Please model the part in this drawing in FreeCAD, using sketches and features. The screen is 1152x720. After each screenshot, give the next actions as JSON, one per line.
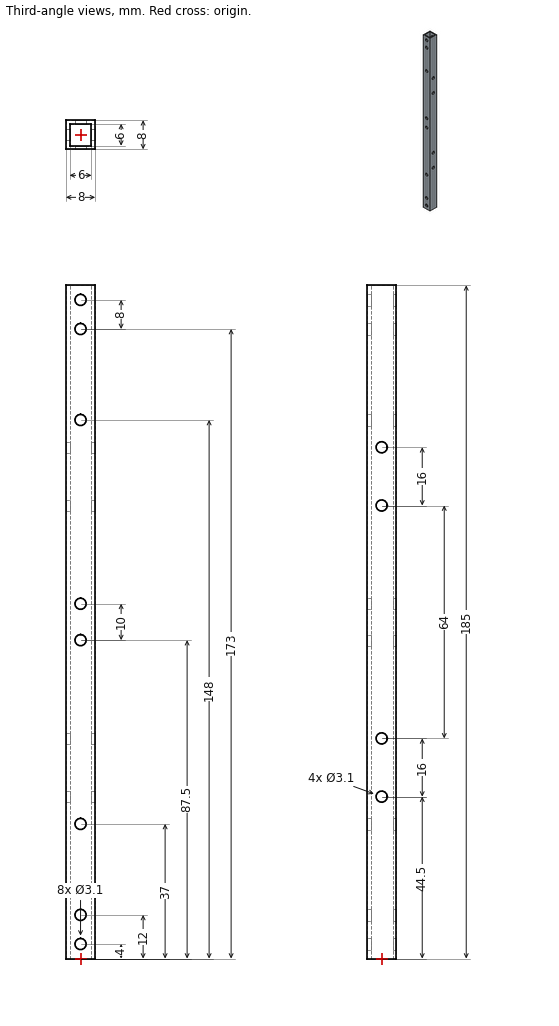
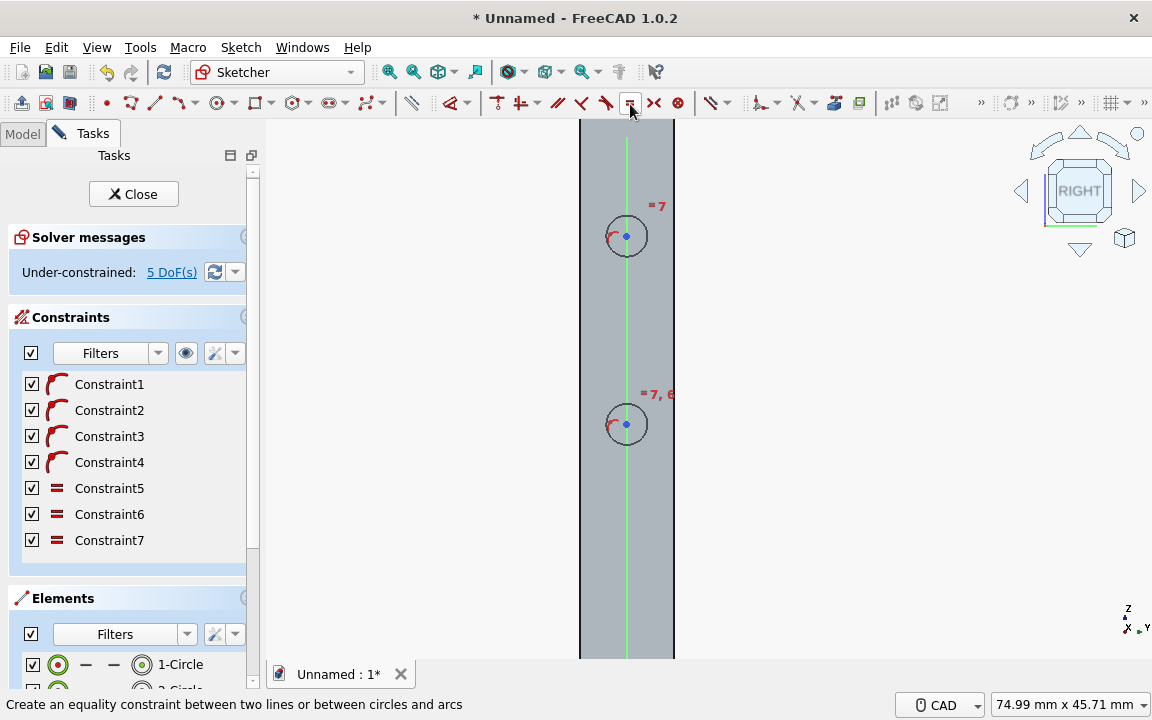
{"action": "left_click", "coordinate": [450, 104]}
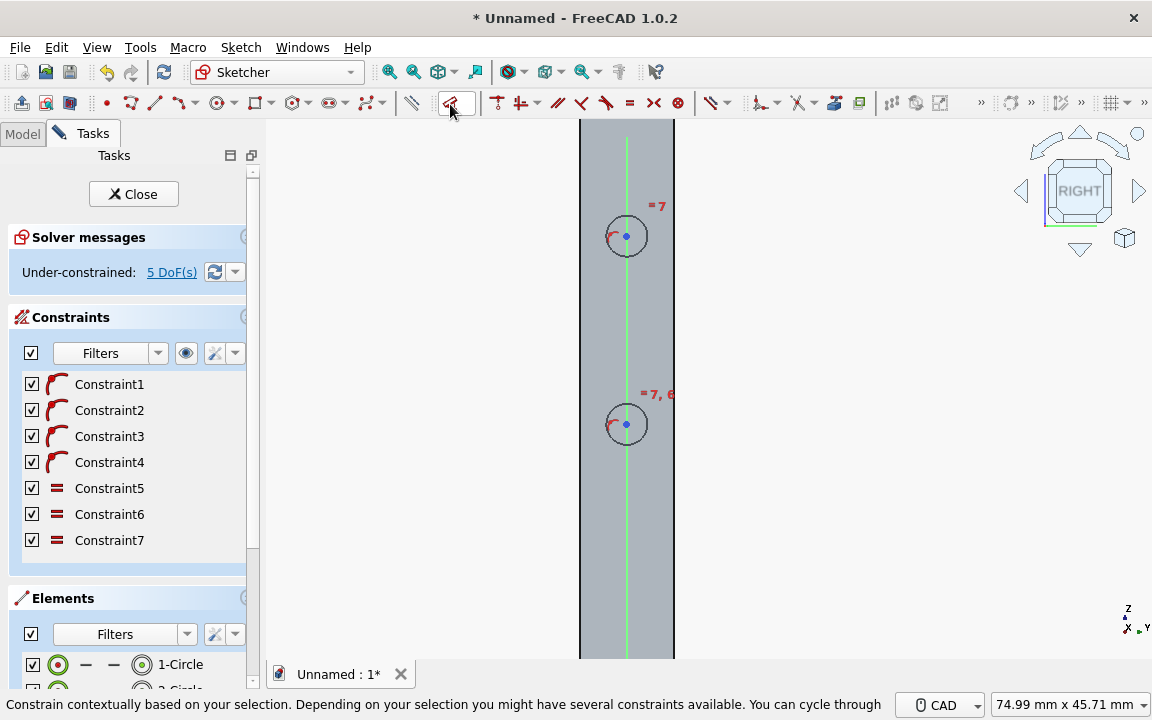
{"action": "scroll", "coordinate": [644, 222], "scroll_direction": "down", "scroll_amount": 8}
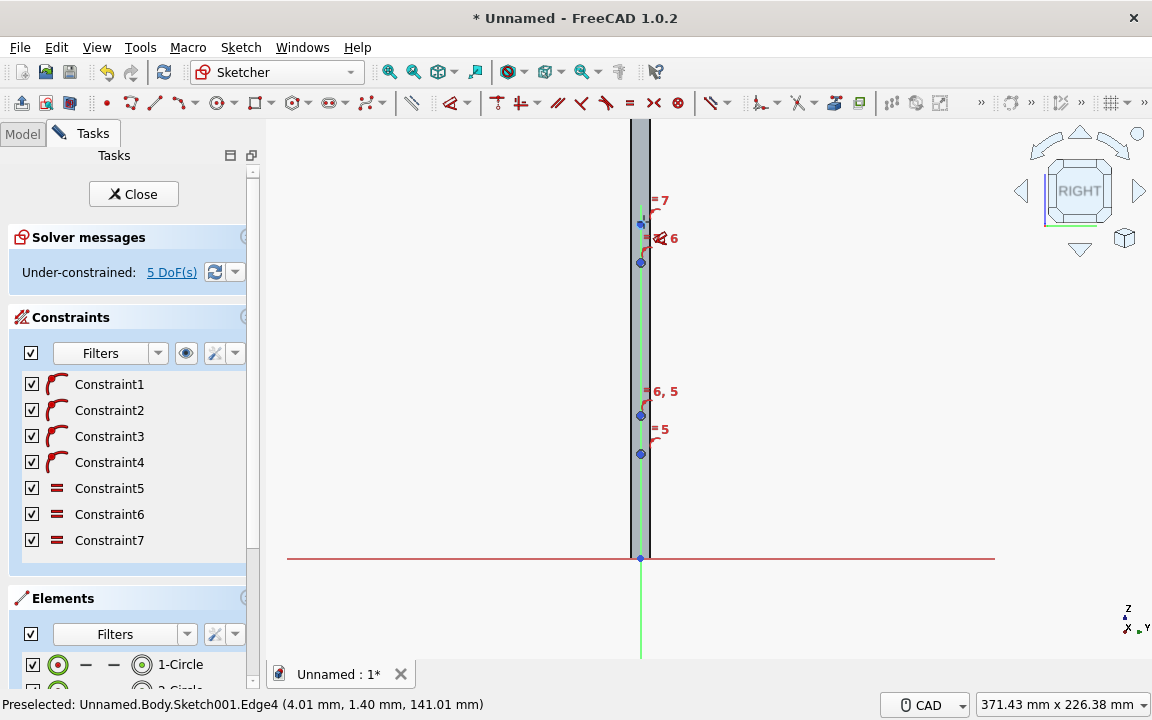
{"action": "scroll", "coordinate": [644, 451], "scroll_direction": "up", "scroll_amount": 9}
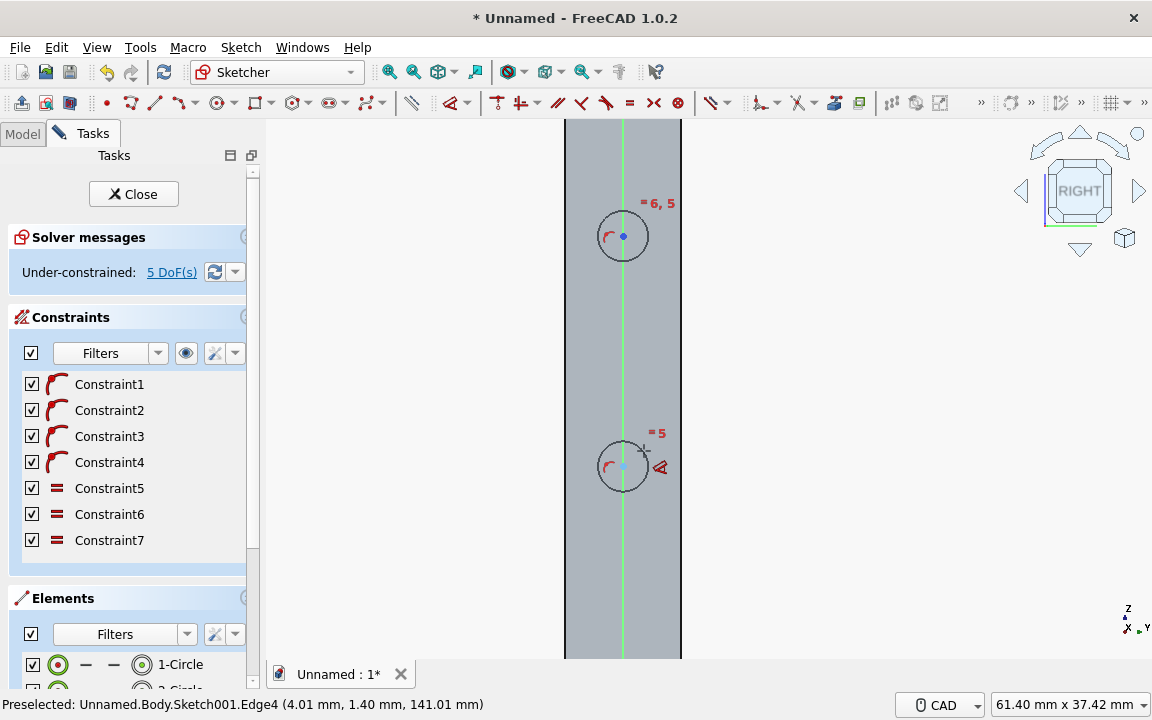
{"action": "left_click", "coordinate": [641, 449]}
{"action": "left_click", "coordinate": [664, 427]}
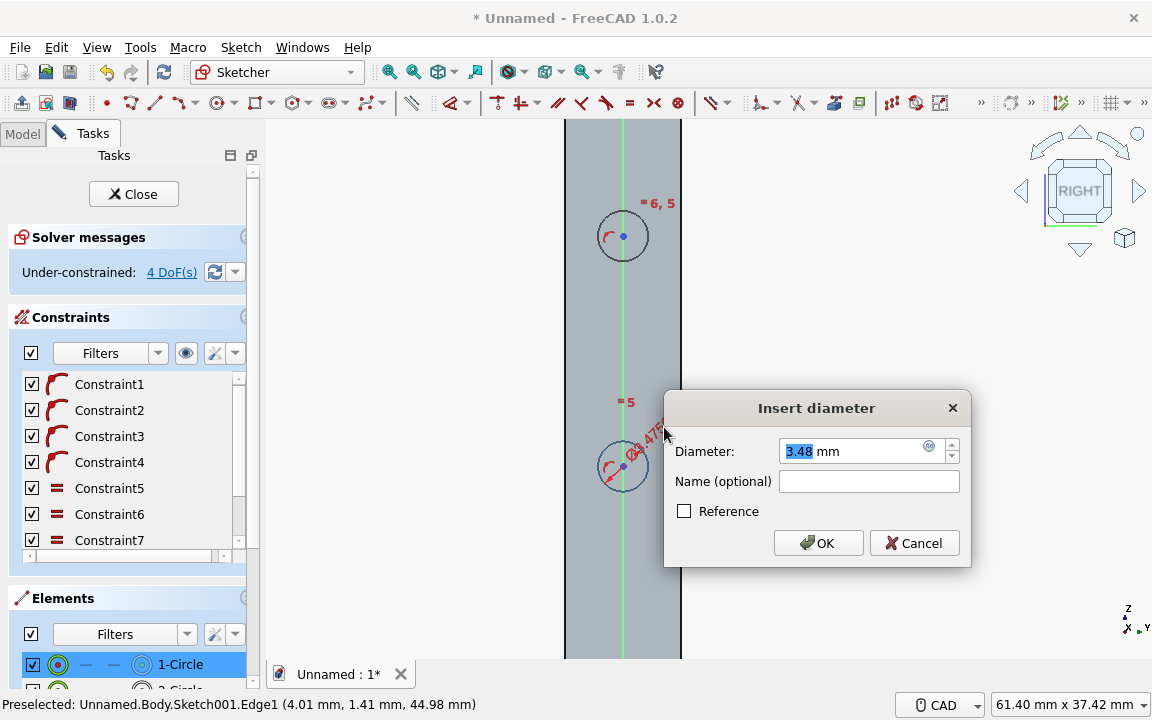
{"action": "type", "text": "3.1"}
{"action": "key", "text": "Return"}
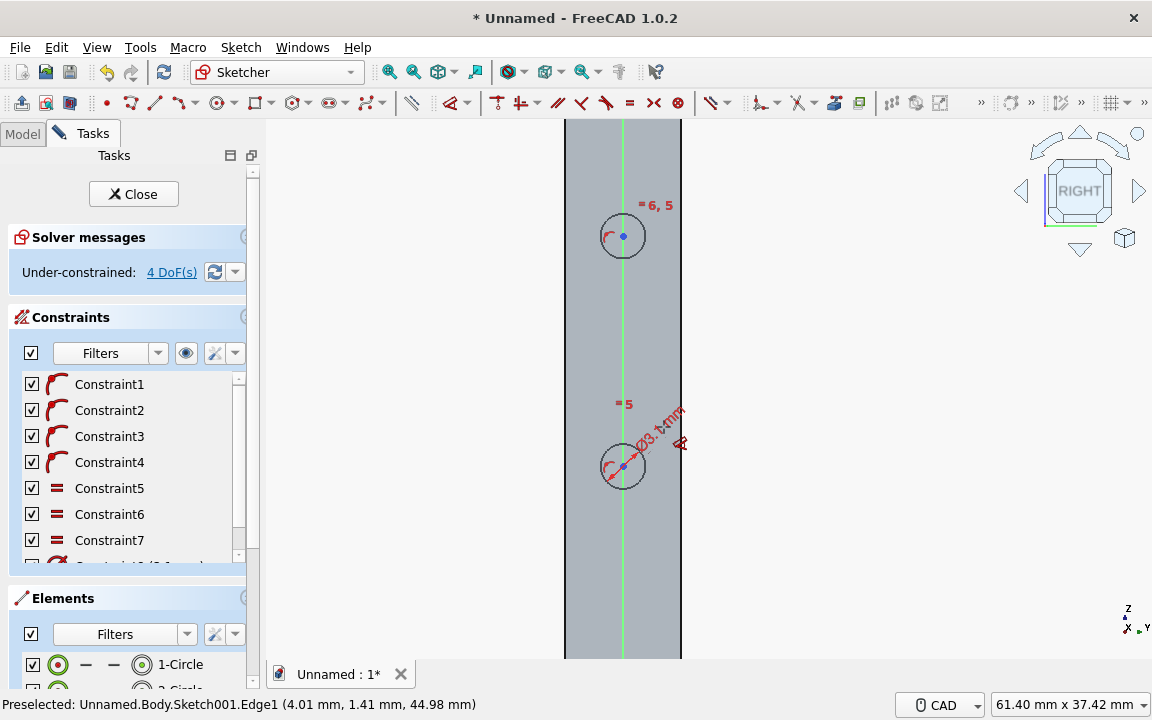
{"action": "scroll", "coordinate": [644, 451], "scroll_direction": "down", "scroll_amount": 9}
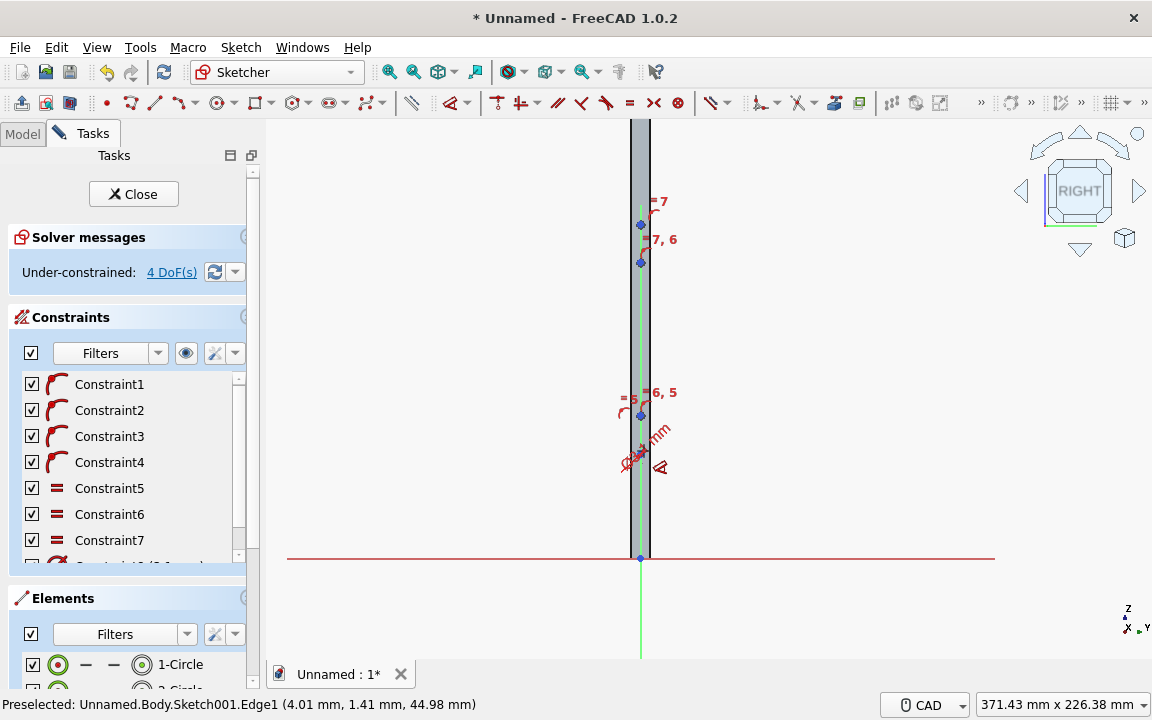
{"action": "left_click", "coordinate": [641, 454]}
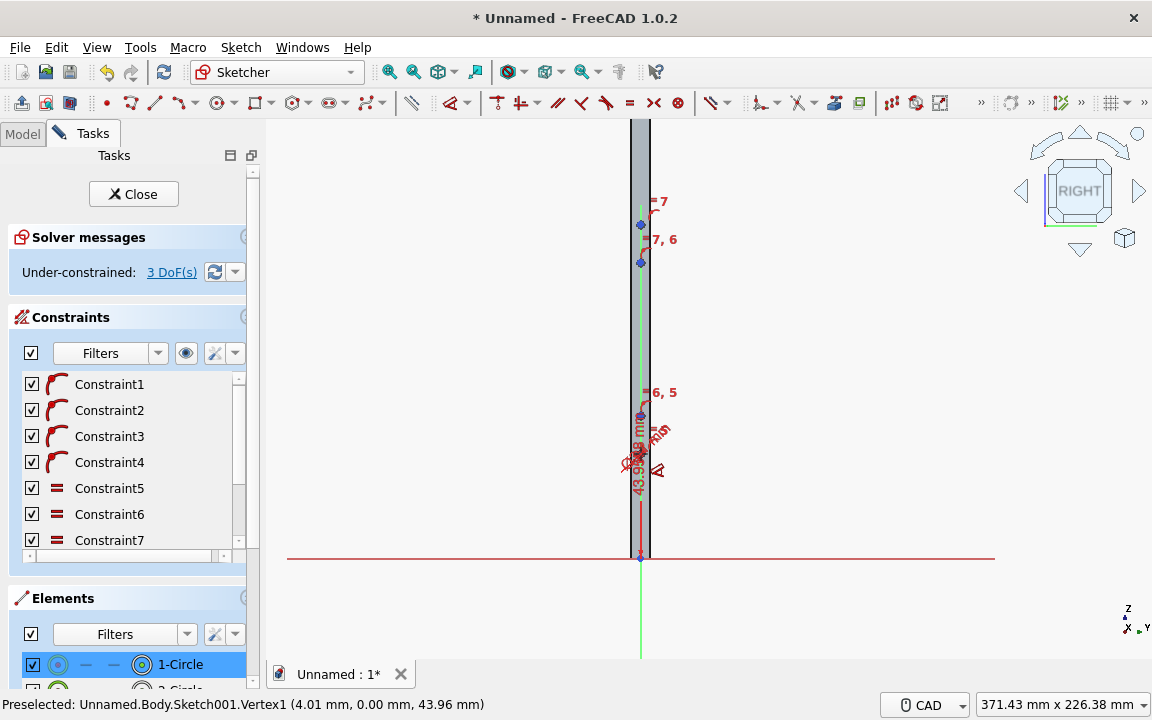
{"action": "left_click", "coordinate": [641, 416]}
{"action": "left_click", "coordinate": [675, 426]}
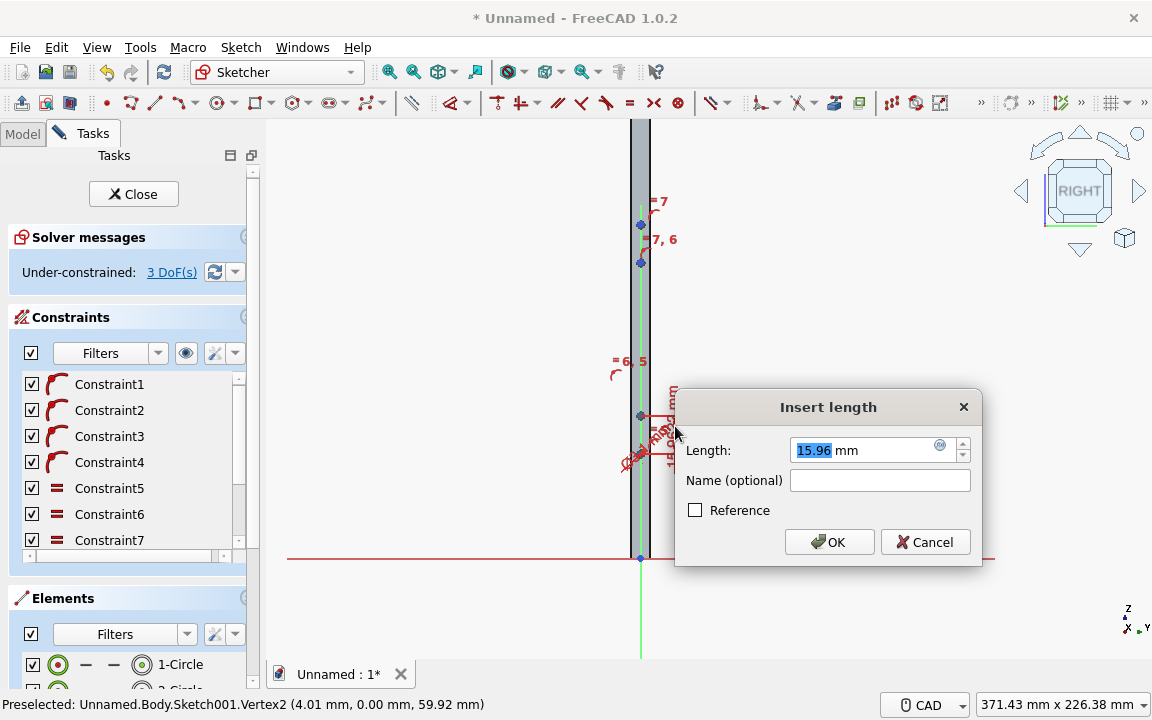
{"action": "type", "text": "16"}
{"action": "key", "text": "Return"}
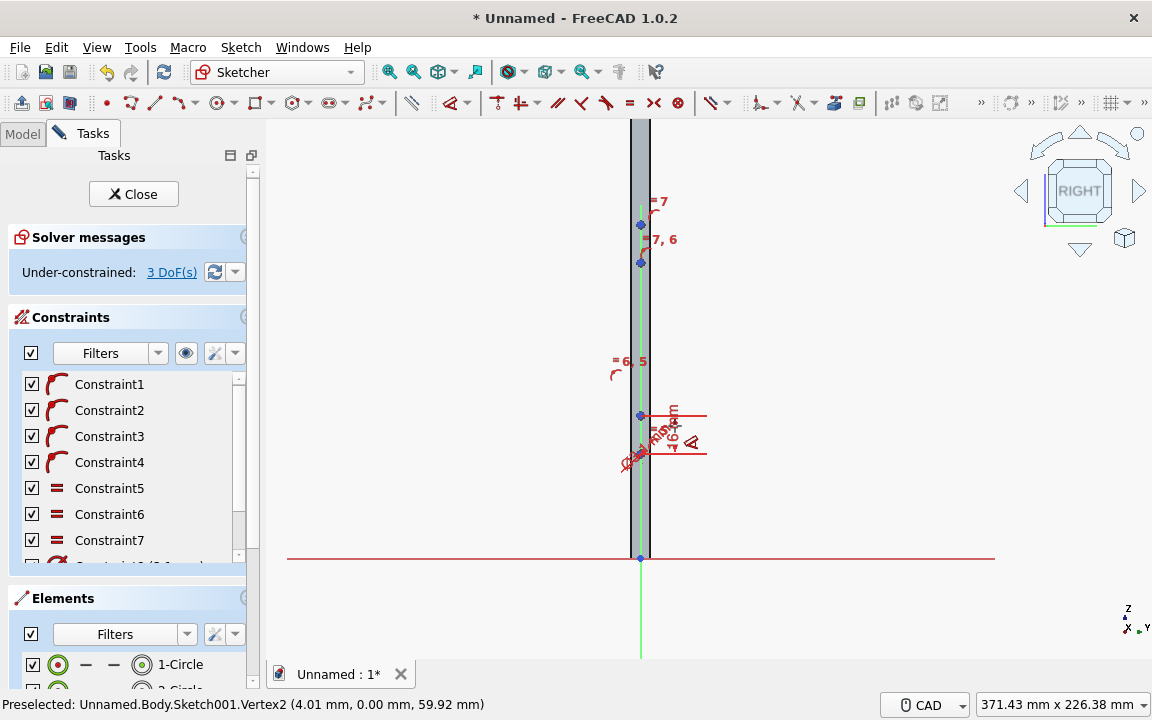
{"action": "left_click", "coordinate": [641, 416]}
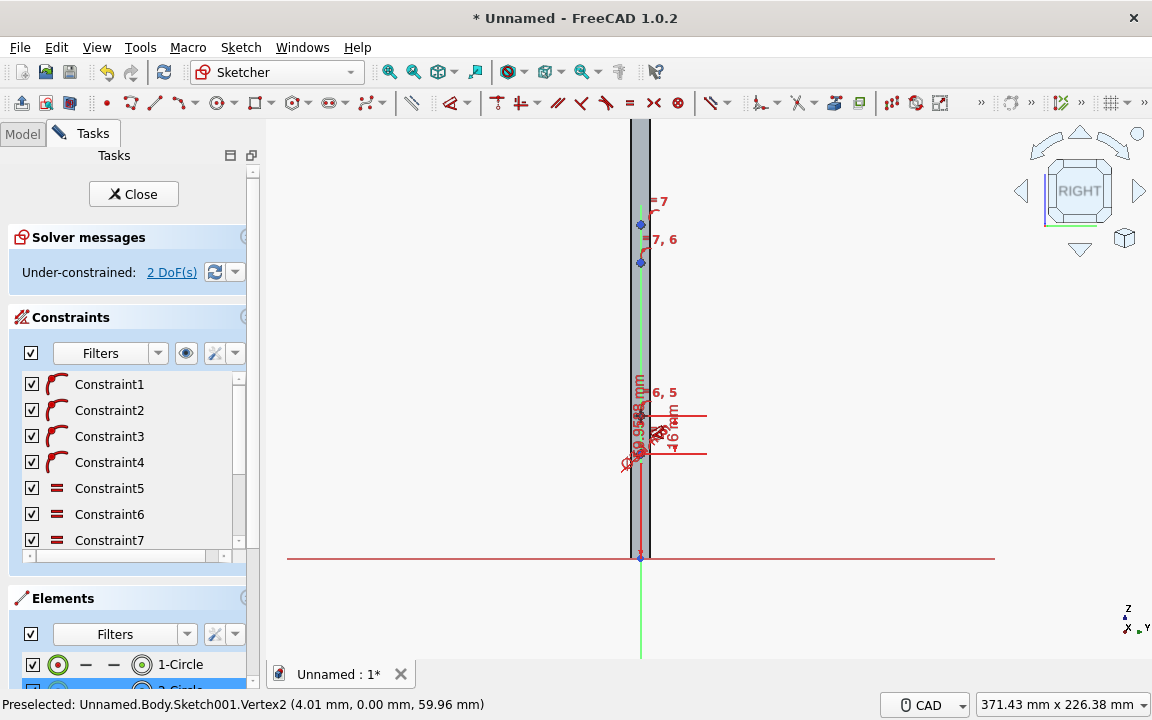
{"action": "left_click", "coordinate": [641, 263]}
{"action": "left_click", "coordinate": [675, 339]}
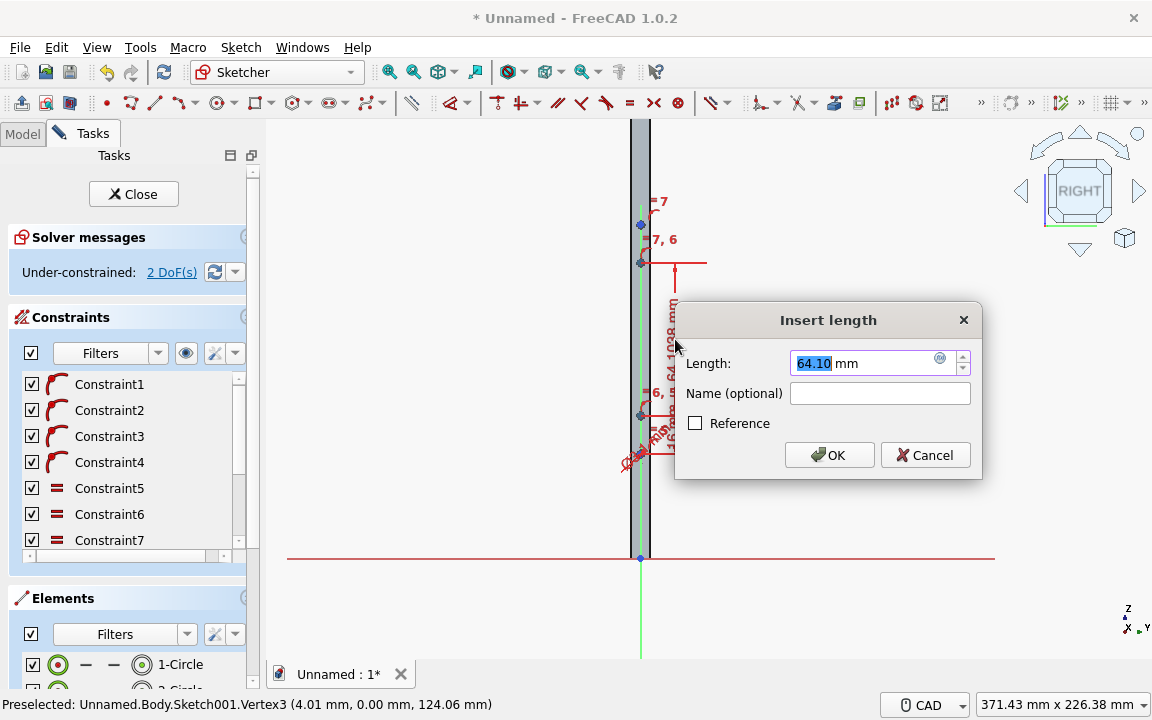
{"action": "type", "text": "64"}
{"action": "key", "text": "Return"}